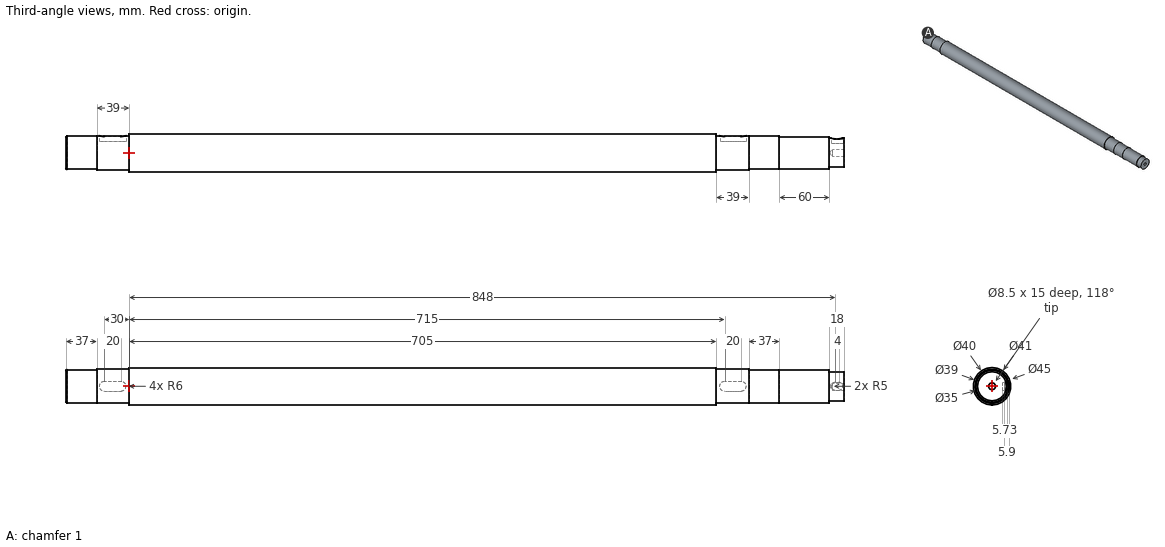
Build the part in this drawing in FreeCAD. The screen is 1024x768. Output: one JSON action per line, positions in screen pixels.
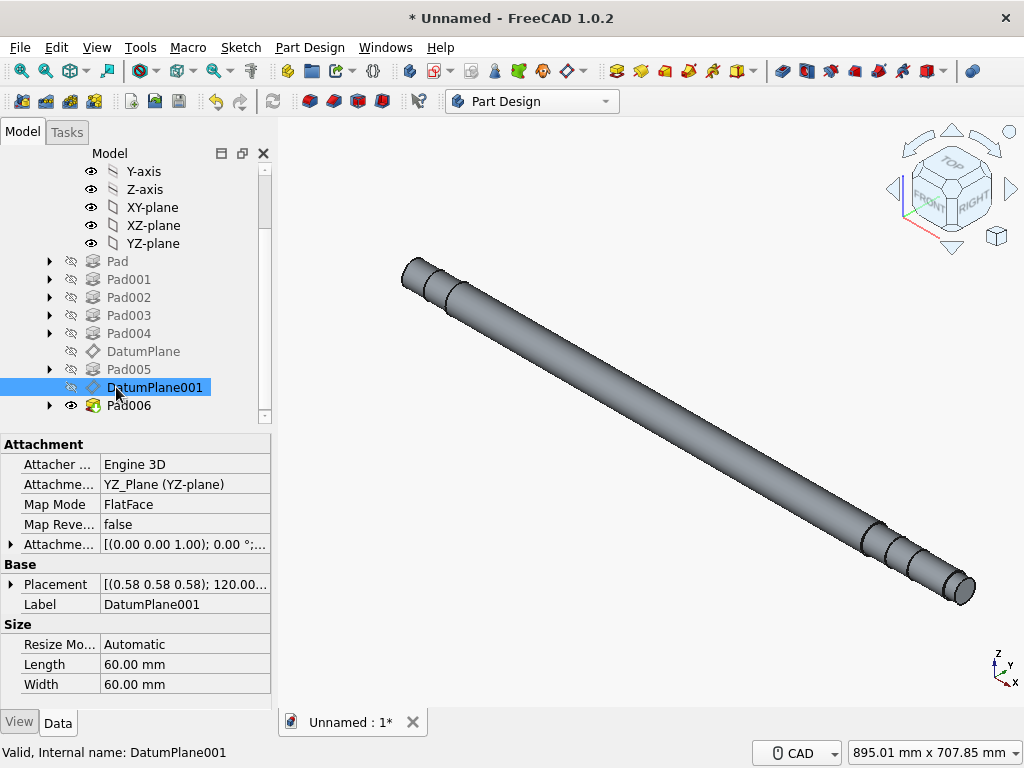
{"action": "left_click", "coordinate": [402, 279]}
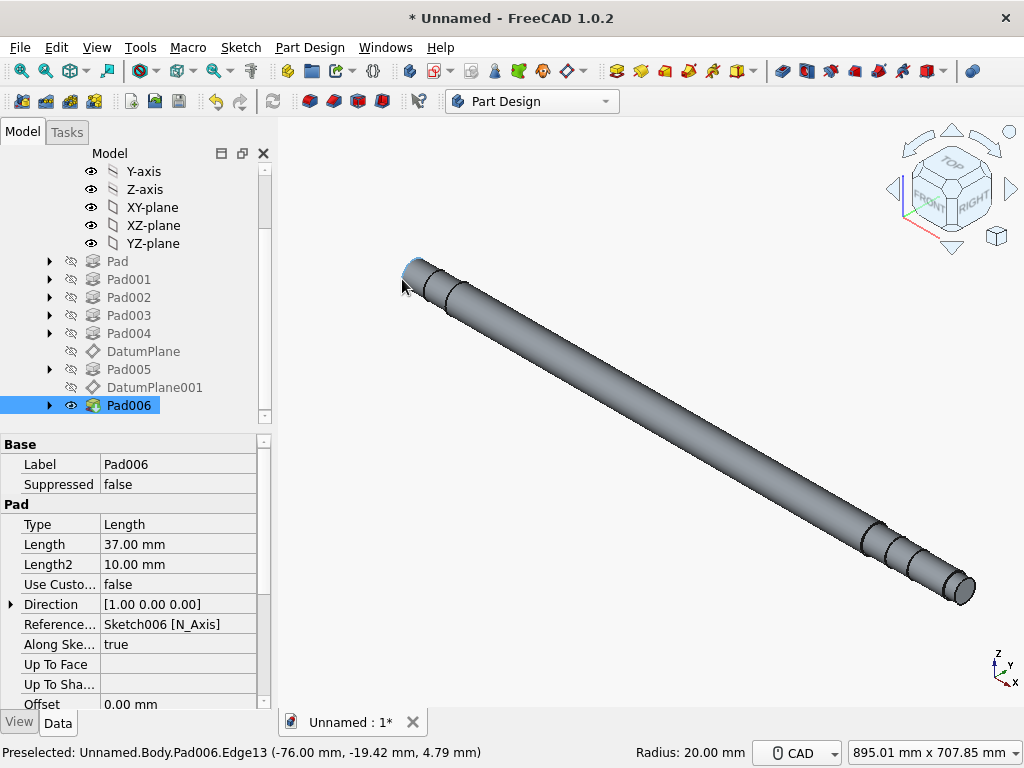
{"action": "left_click", "coordinate": [334, 102]}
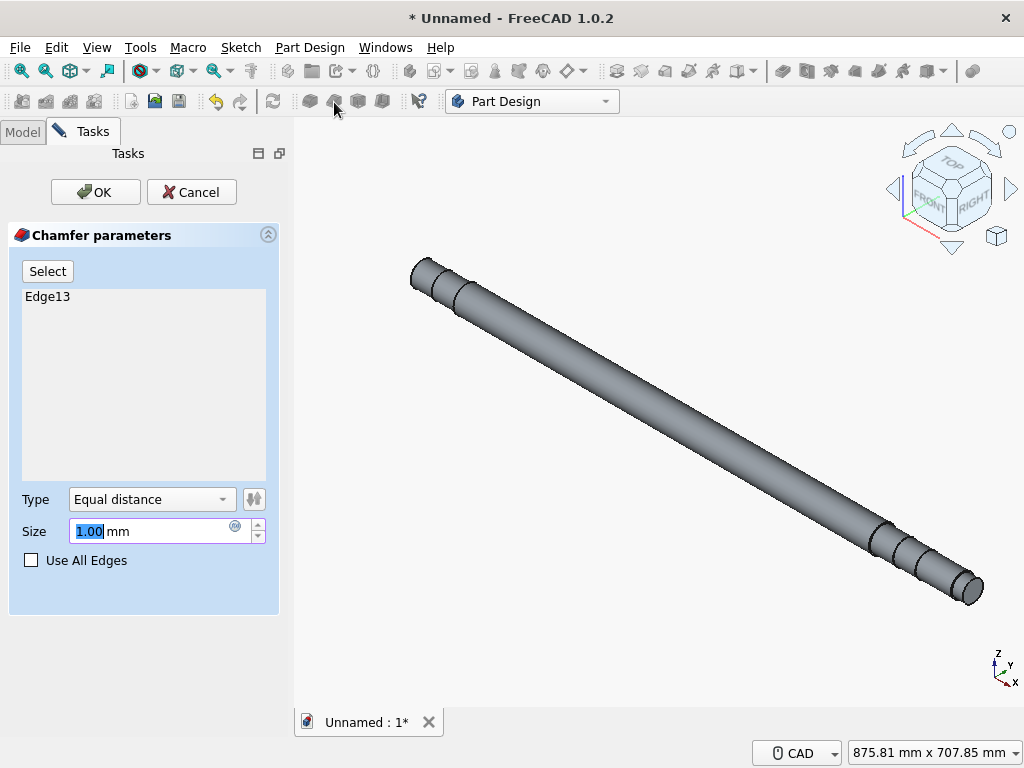
{"action": "type", "text": "1"}
{"action": "key", "text": "Tab"}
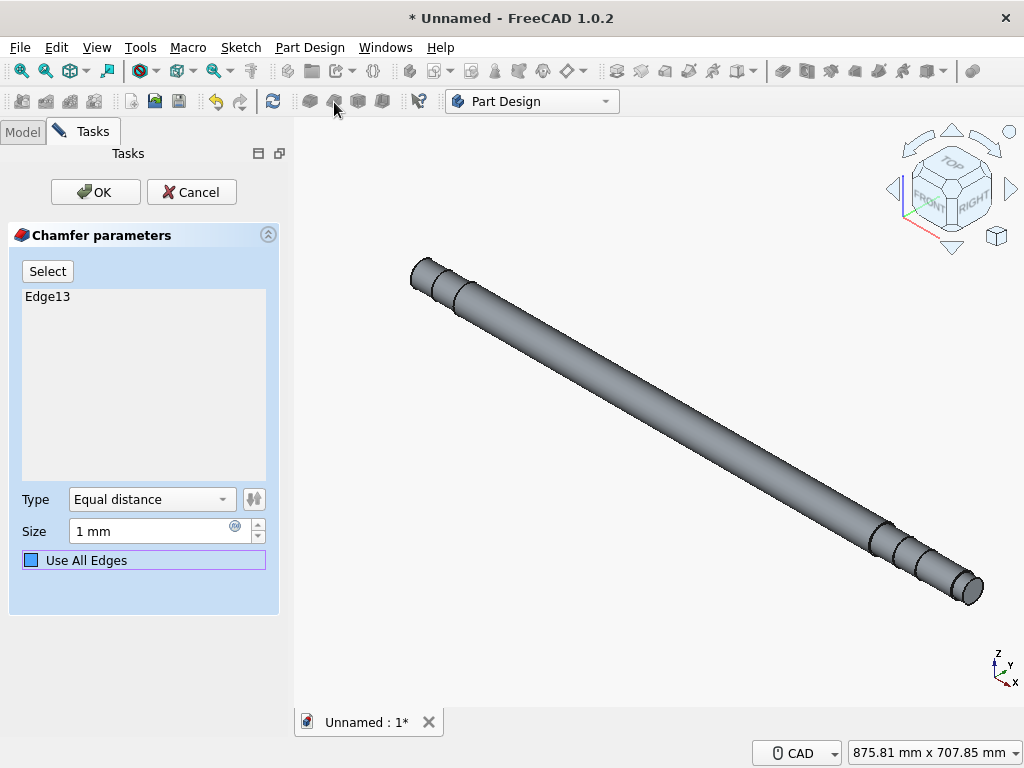
{"action": "left_click", "coordinate": [96, 192]}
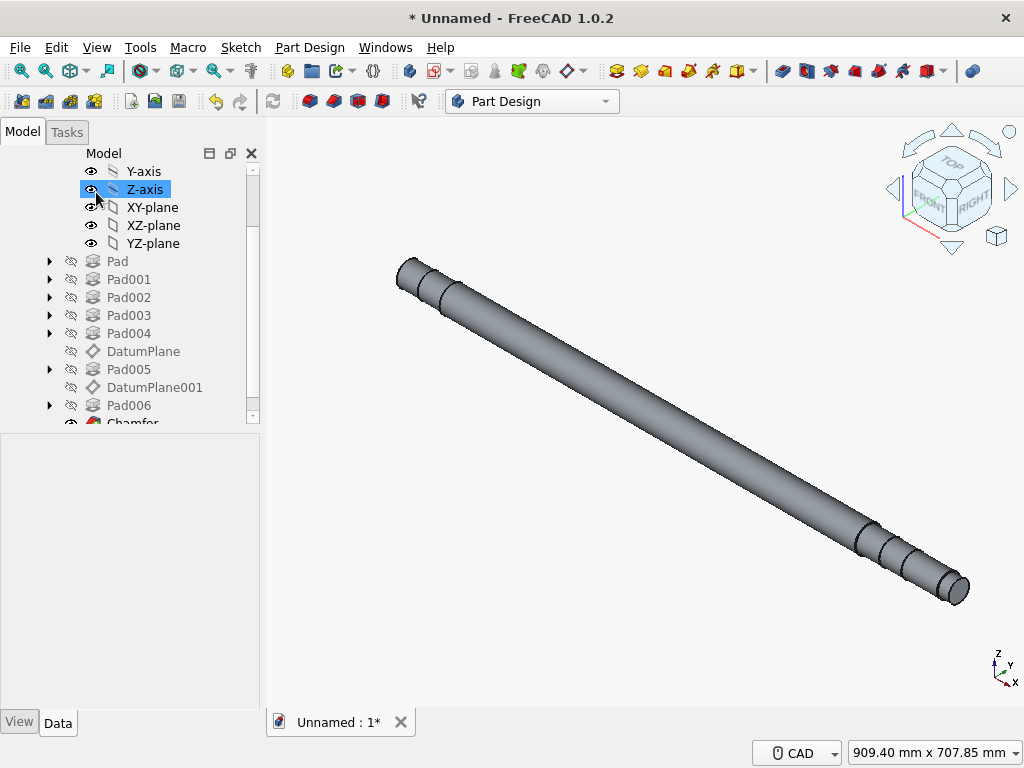
{"action": "scroll", "coordinate": [160, 293], "scroll_direction": "down", "scroll_amount": 3}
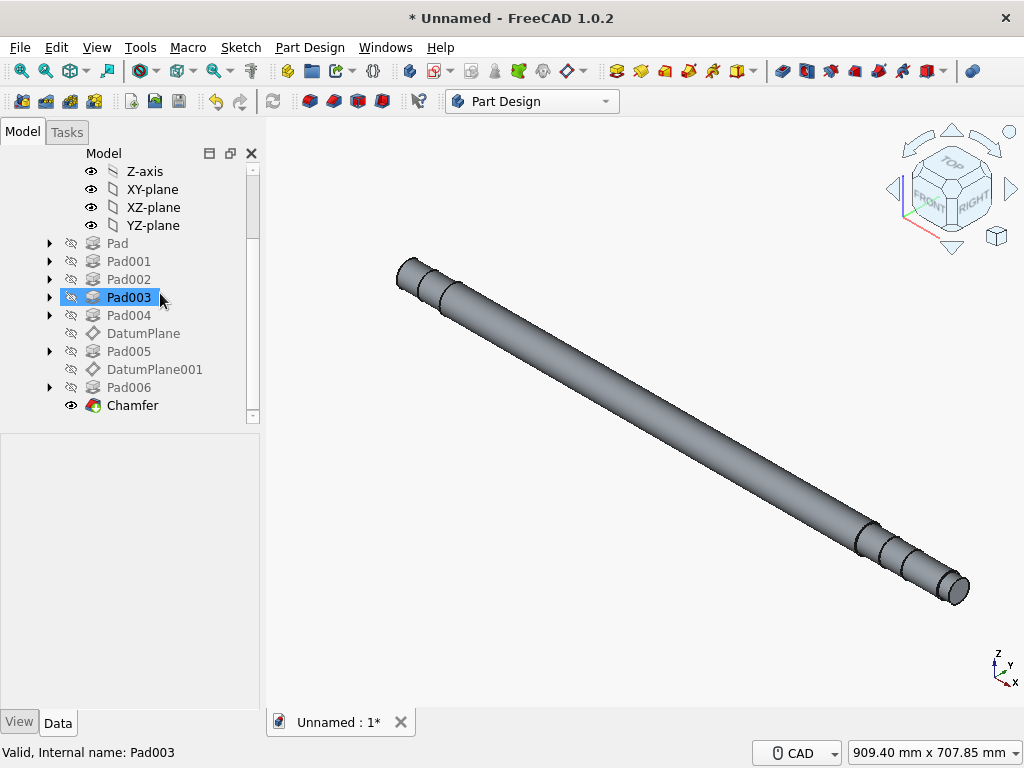
{"action": "scroll", "coordinate": [160, 293], "scroll_direction": "up", "scroll_amount": 15}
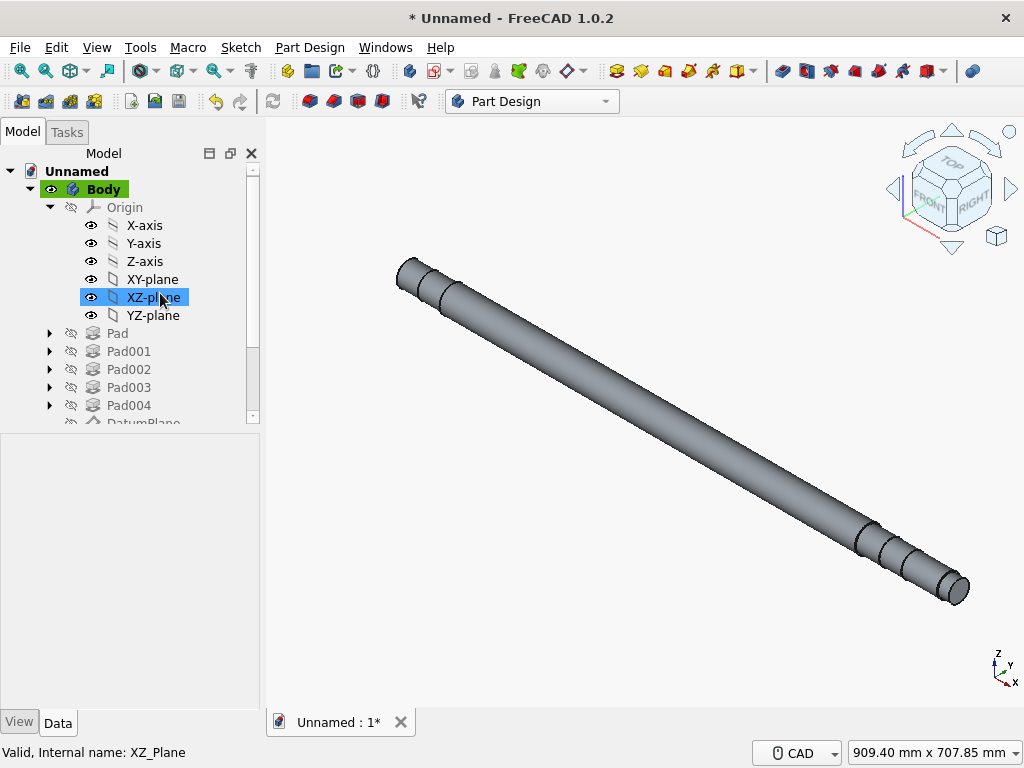
{"action": "left_click", "coordinate": [136, 297]}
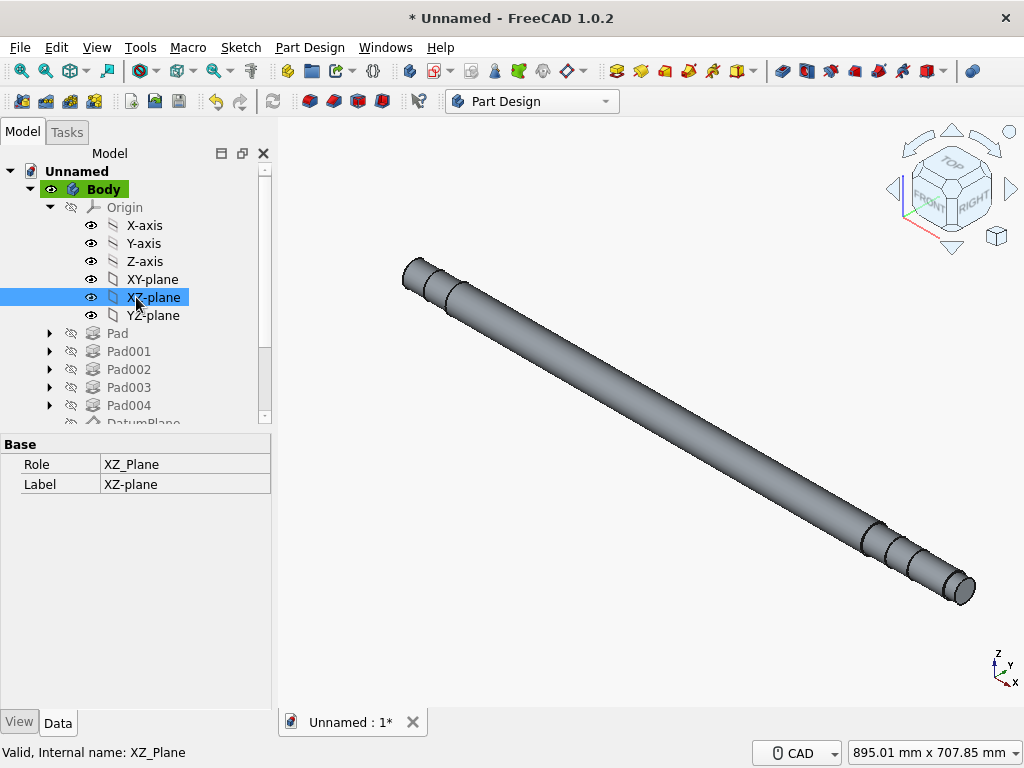
{"action": "left_click", "coordinate": [568, 72]}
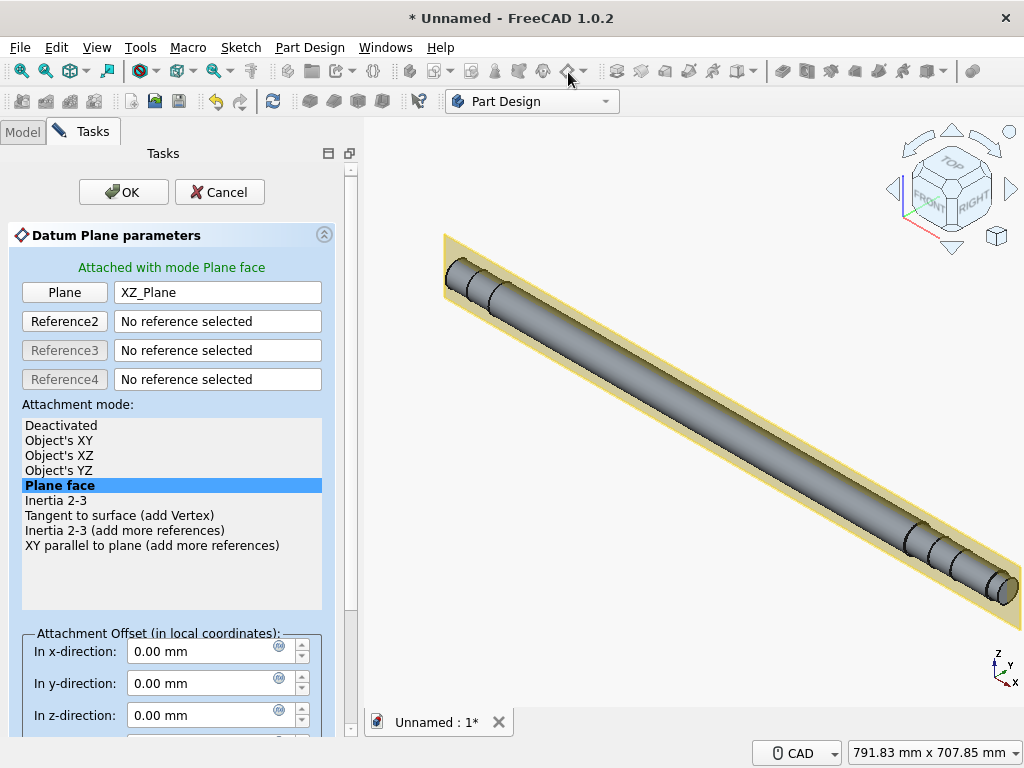
{"action": "triple_click", "coordinate": [210, 715]}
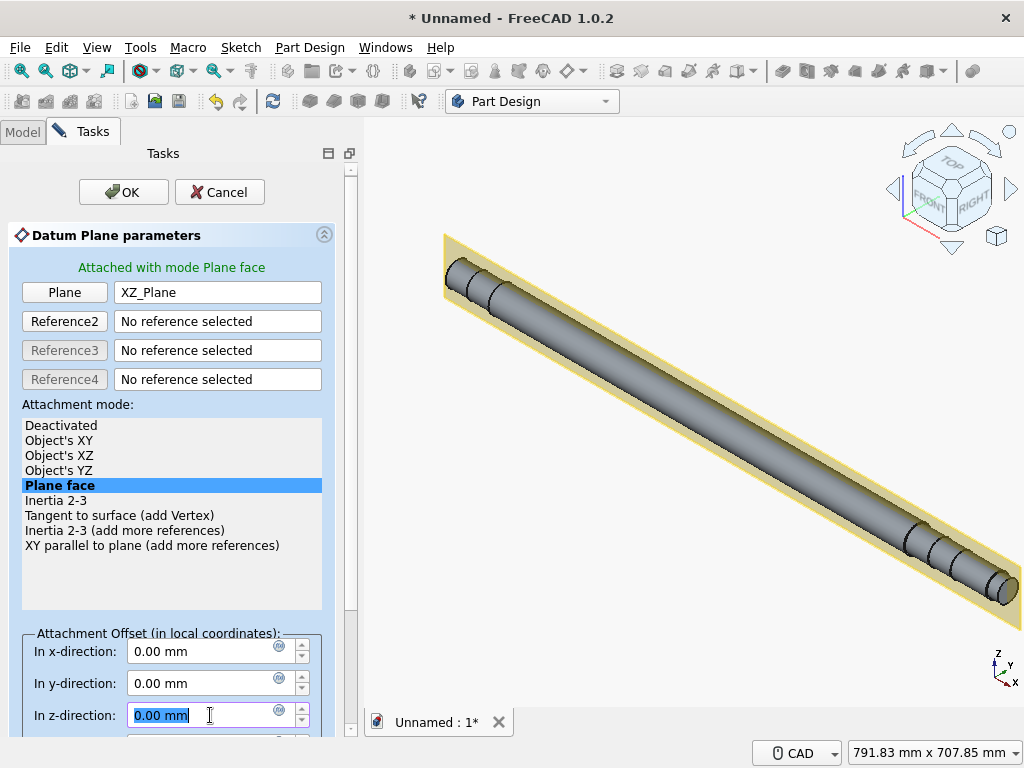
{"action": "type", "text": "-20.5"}
{"action": "key", "text": "Tab"}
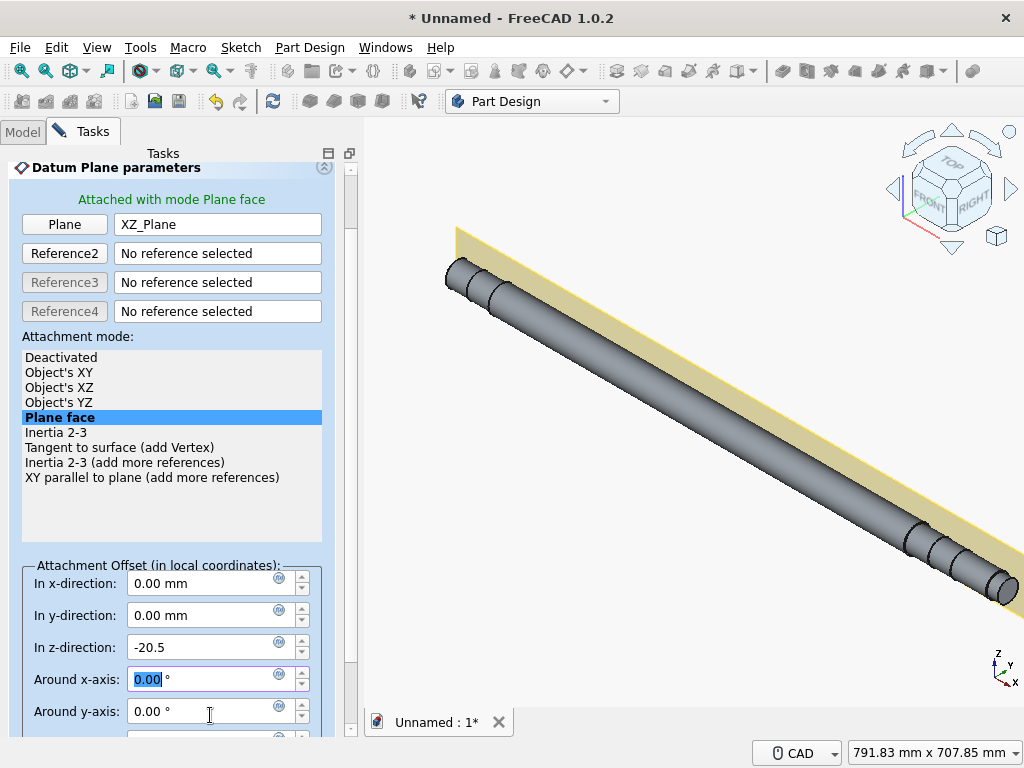
{"action": "scroll", "coordinate": [351, 450], "scroll_direction": "up", "scroll_amount": 2}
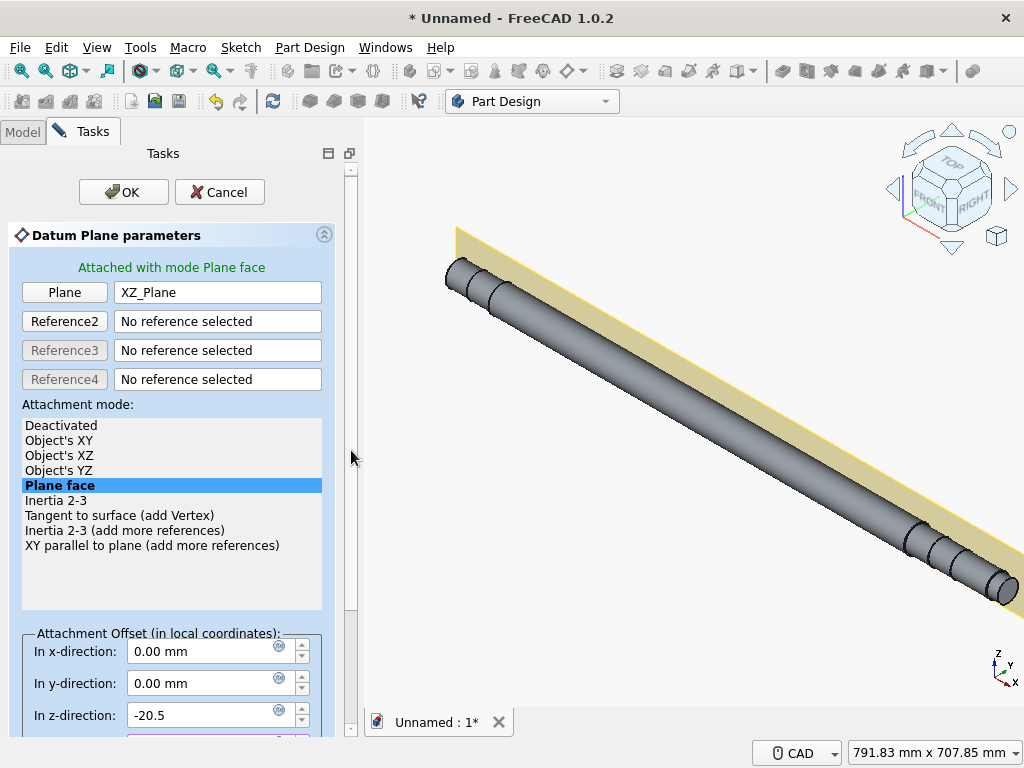
{"action": "left_click", "coordinate": [124, 192]}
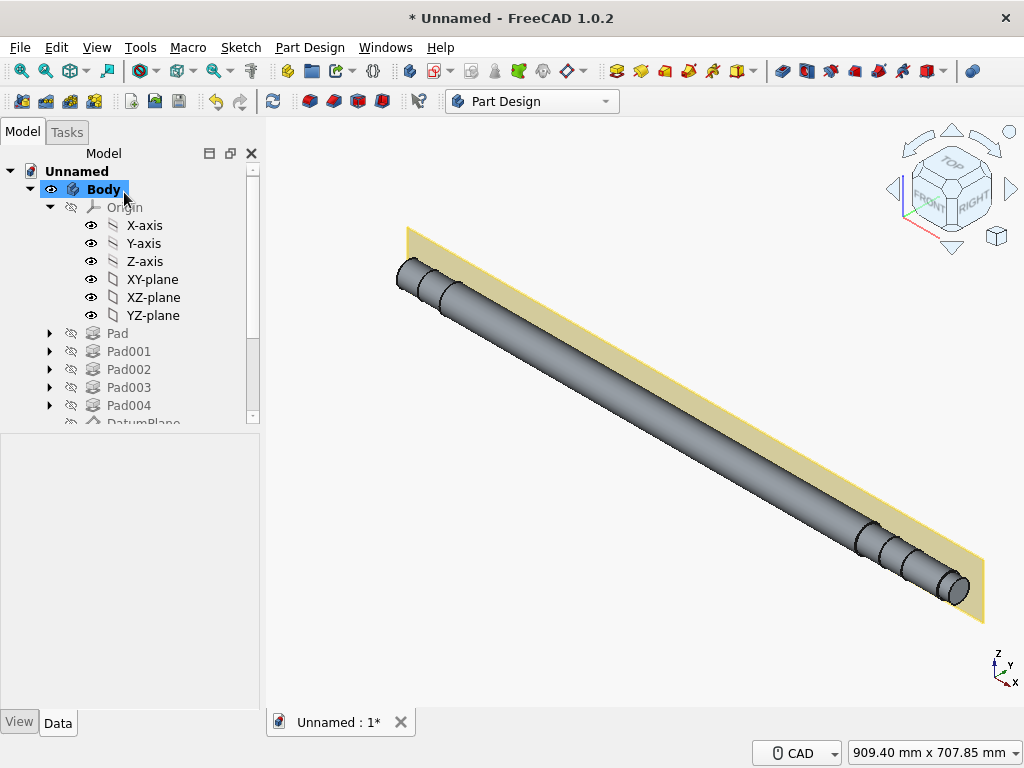
{"action": "scroll", "coordinate": [100, 293], "scroll_direction": "down", "scroll_amount": 3}